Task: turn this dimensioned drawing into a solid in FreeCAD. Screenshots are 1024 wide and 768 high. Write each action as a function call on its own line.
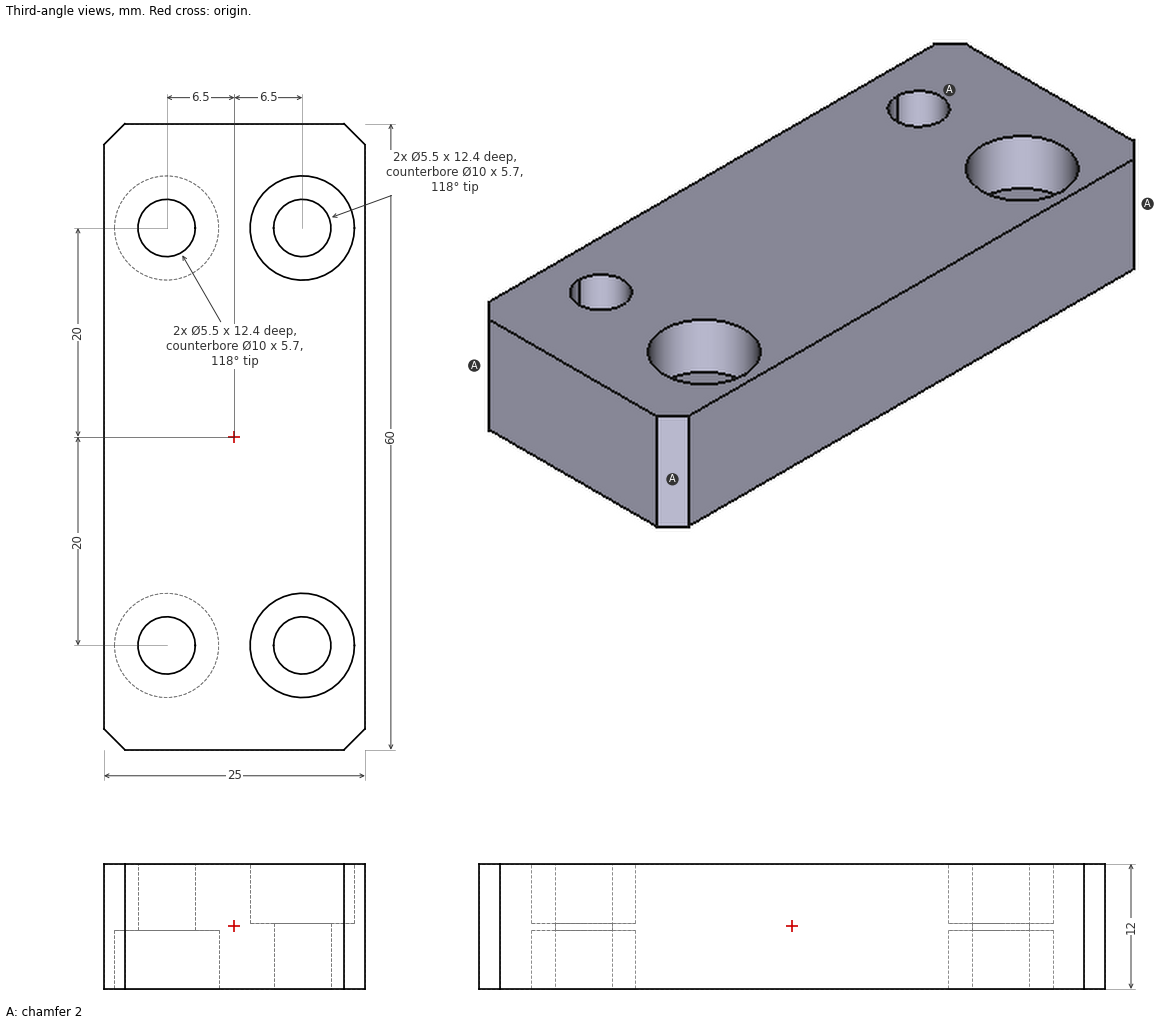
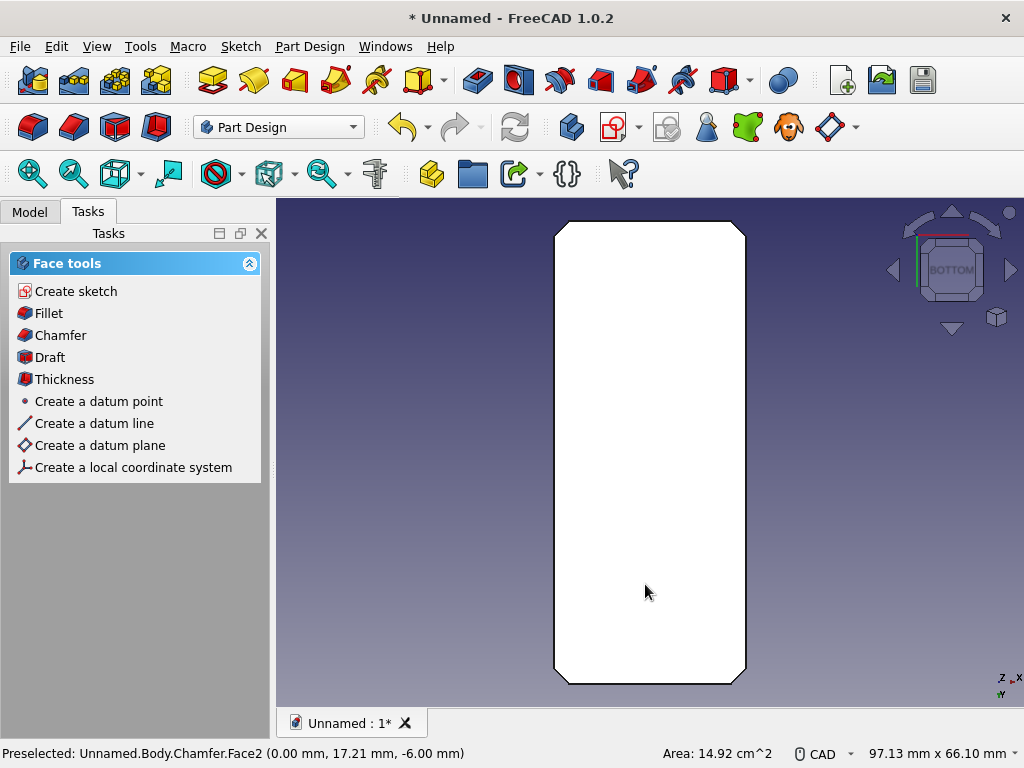
click(612, 128)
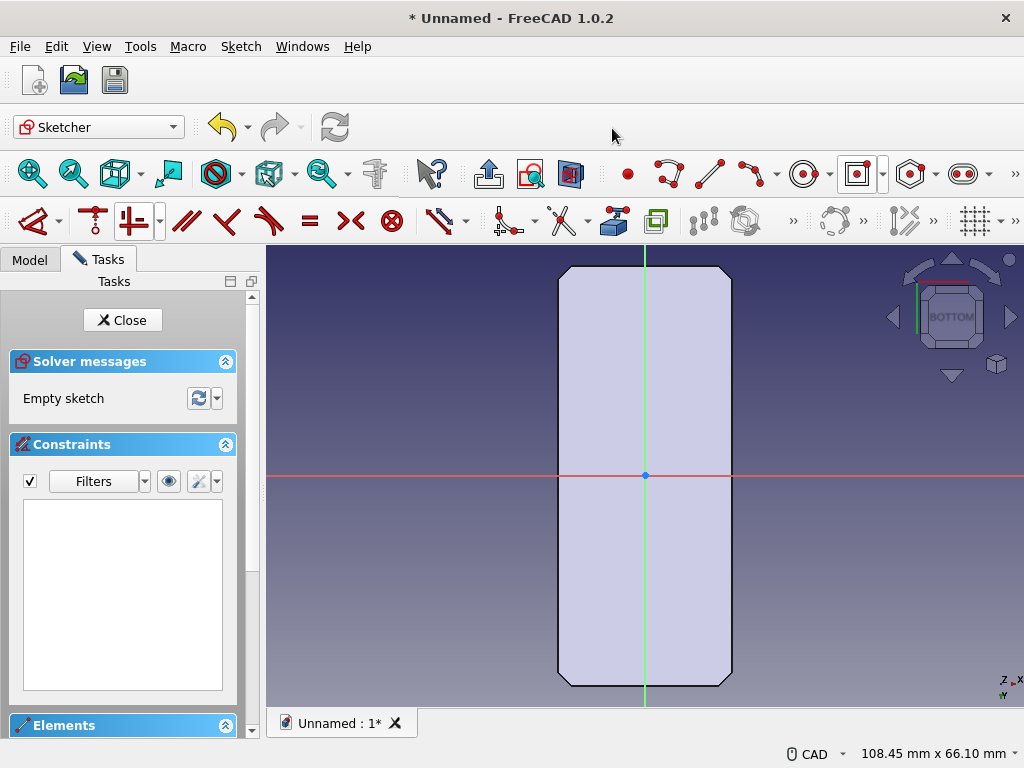
click(804, 174)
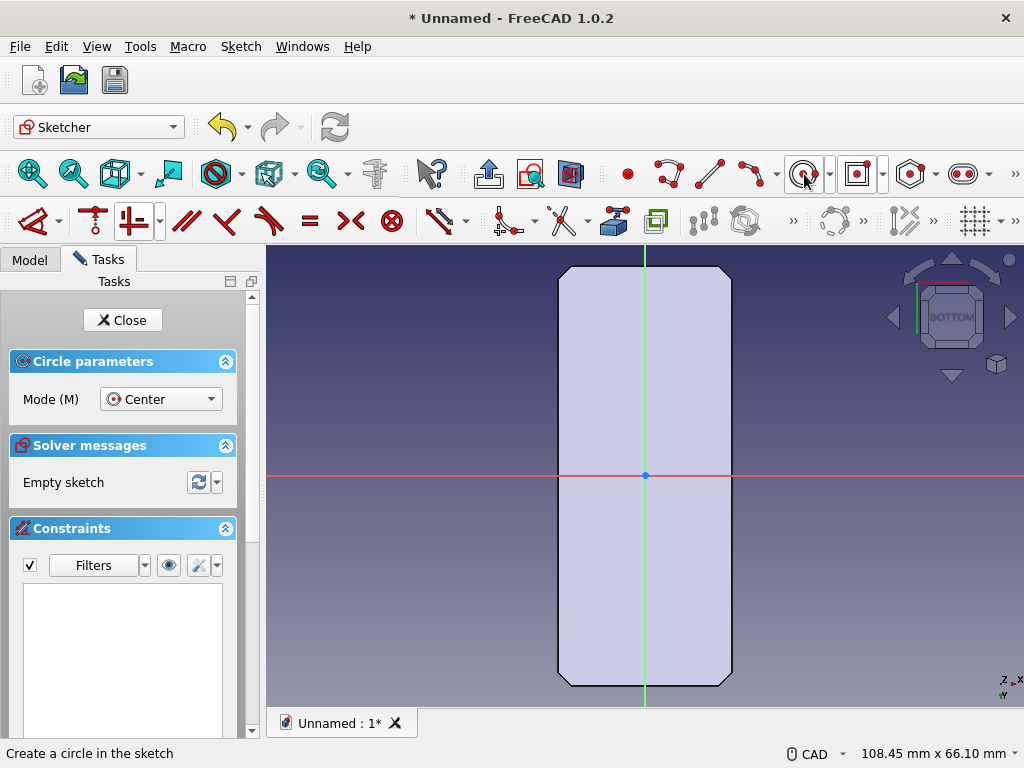
click(600, 616)
click(613, 602)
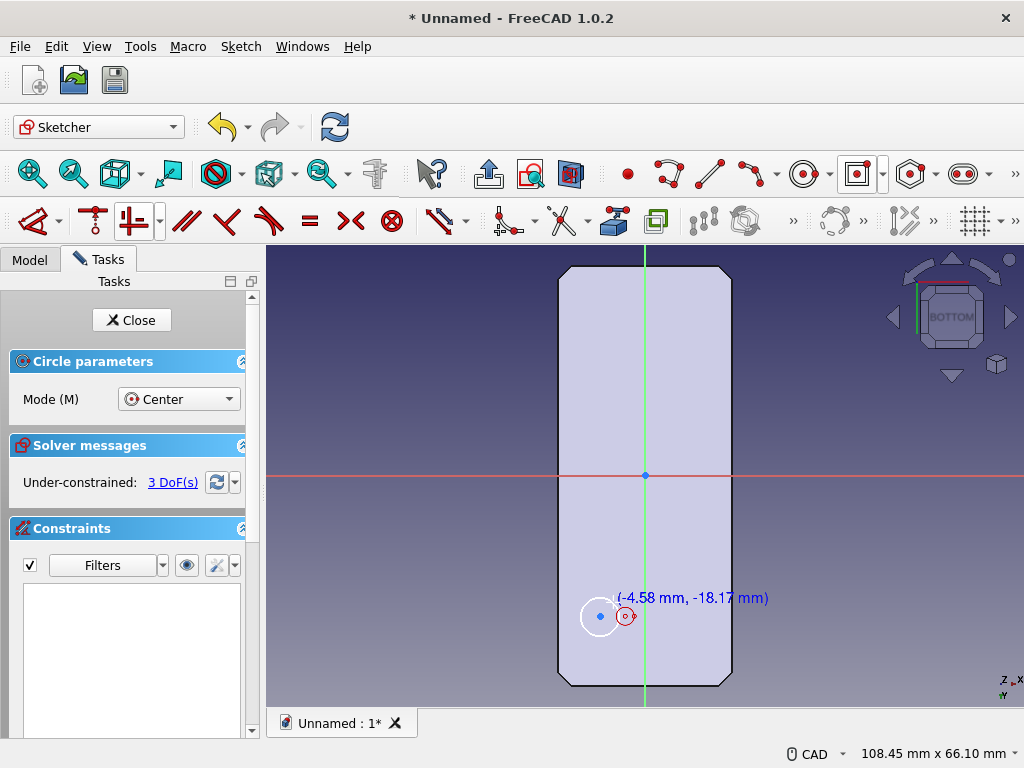
click(600, 336)
click(613, 323)
key(Escape)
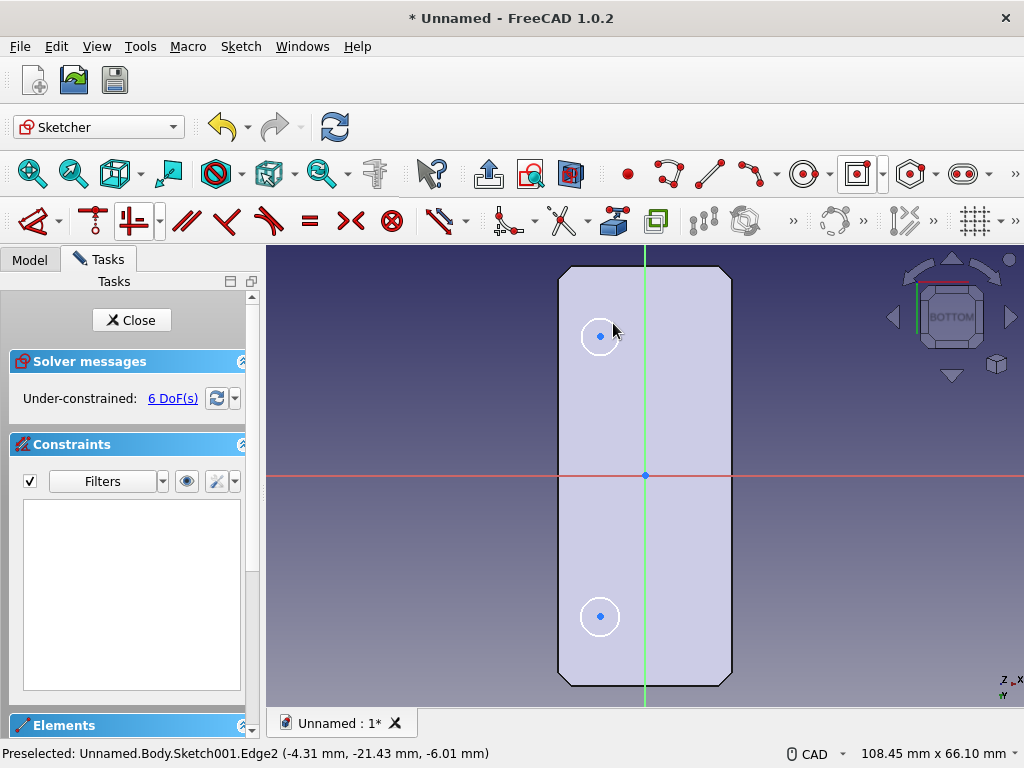
click(613, 603)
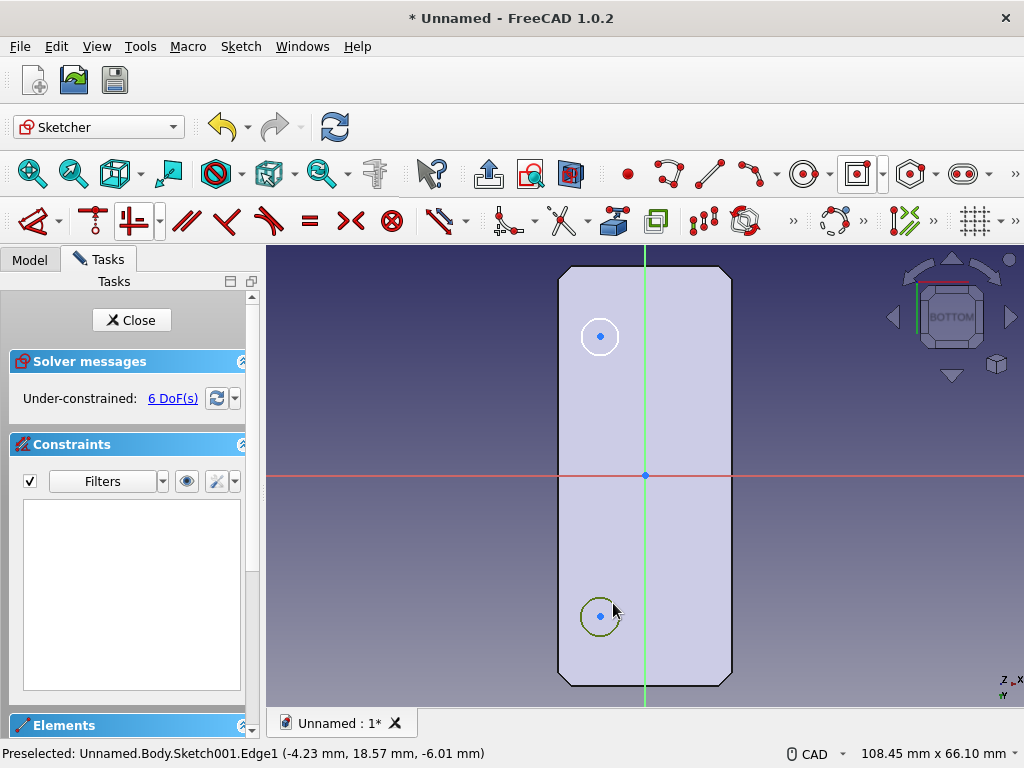
click(613, 324)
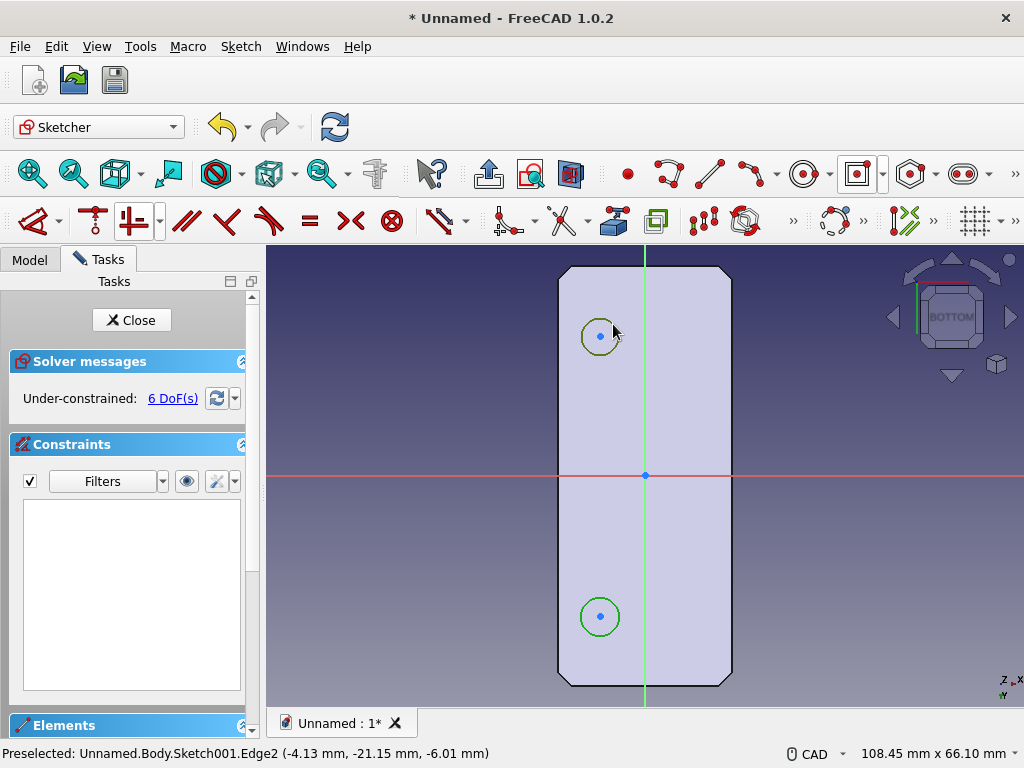
click(310, 222)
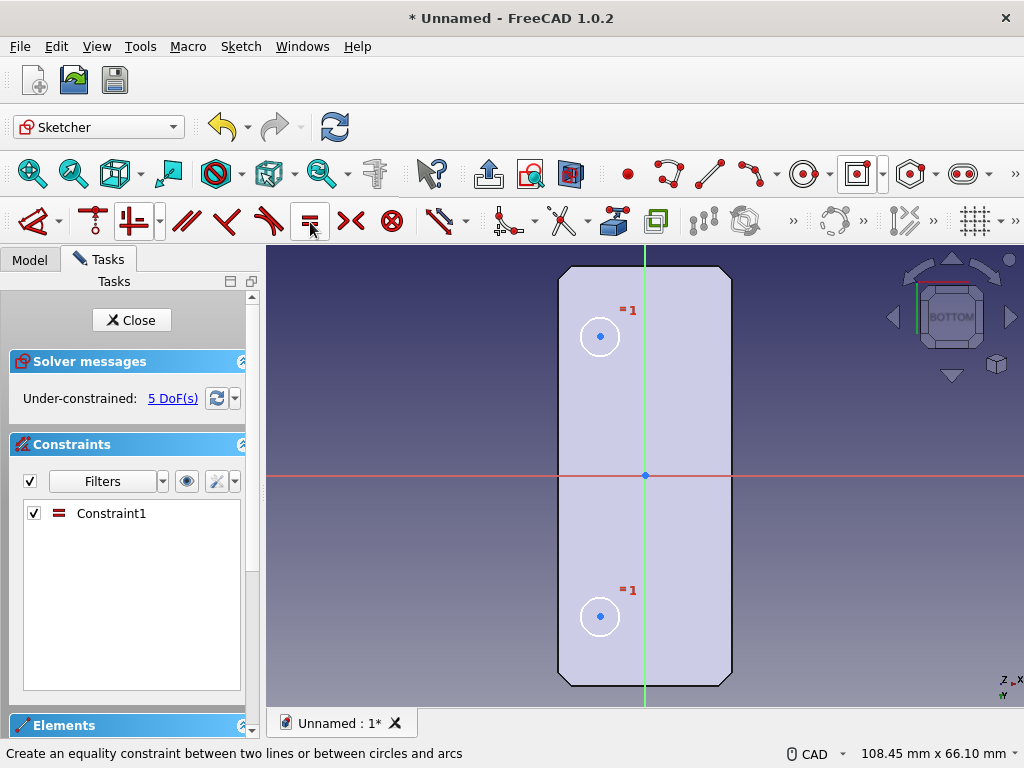
click(600, 617)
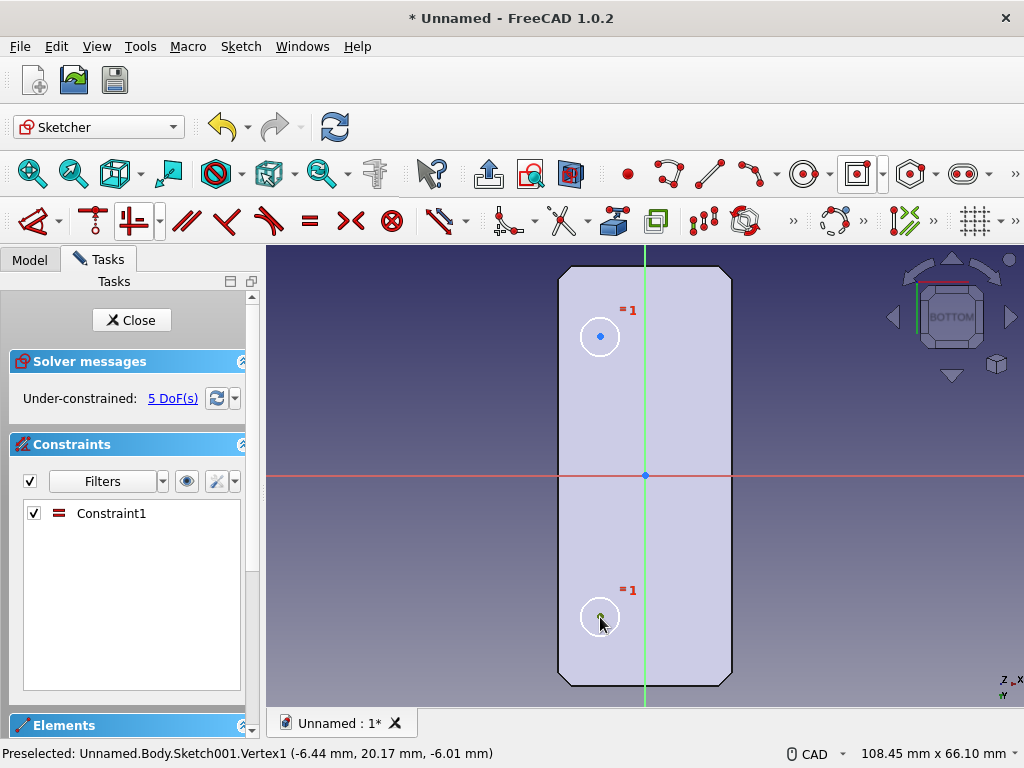
click(600, 337)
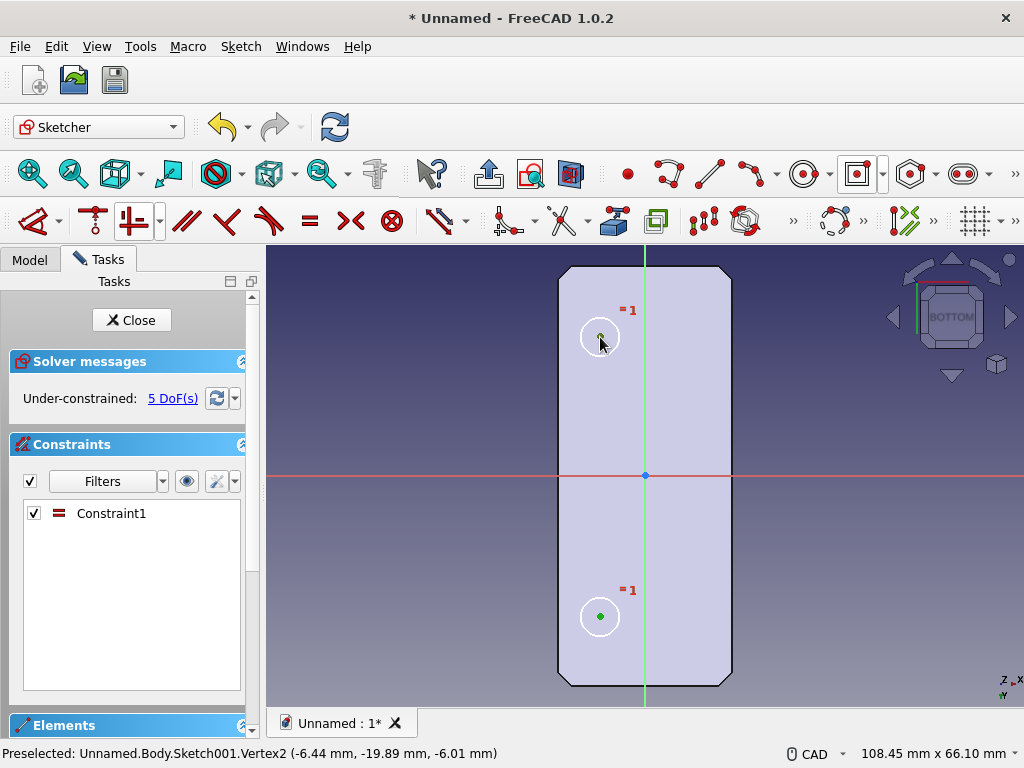
click(160, 222)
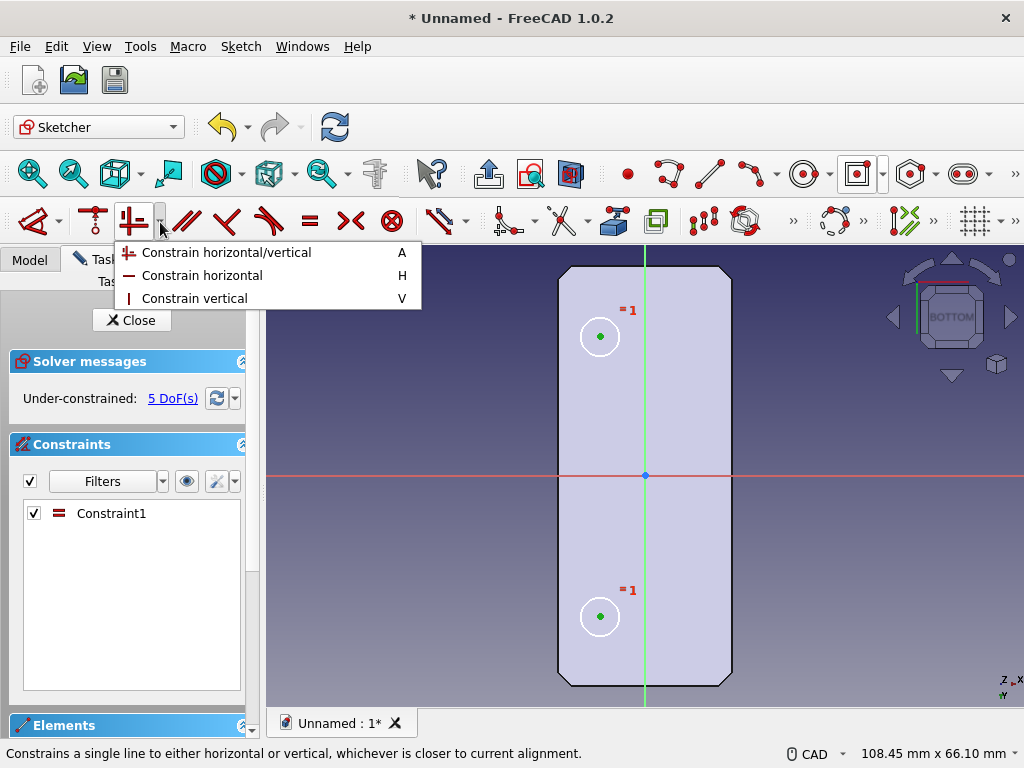
click(268, 298)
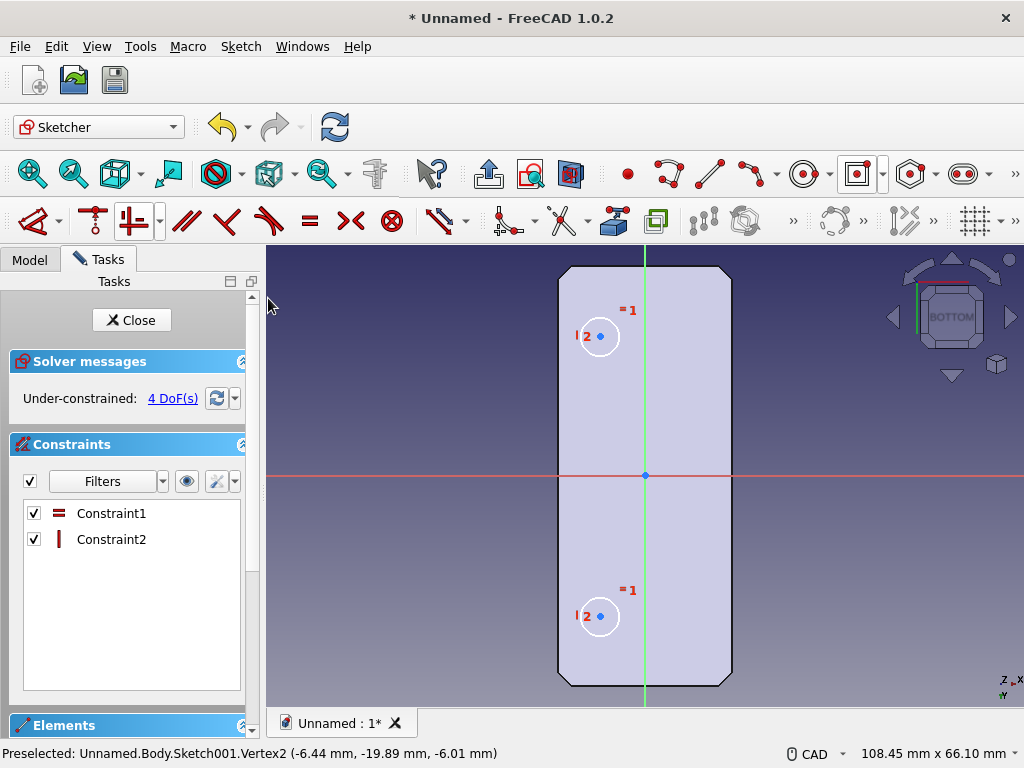
click(32, 222)